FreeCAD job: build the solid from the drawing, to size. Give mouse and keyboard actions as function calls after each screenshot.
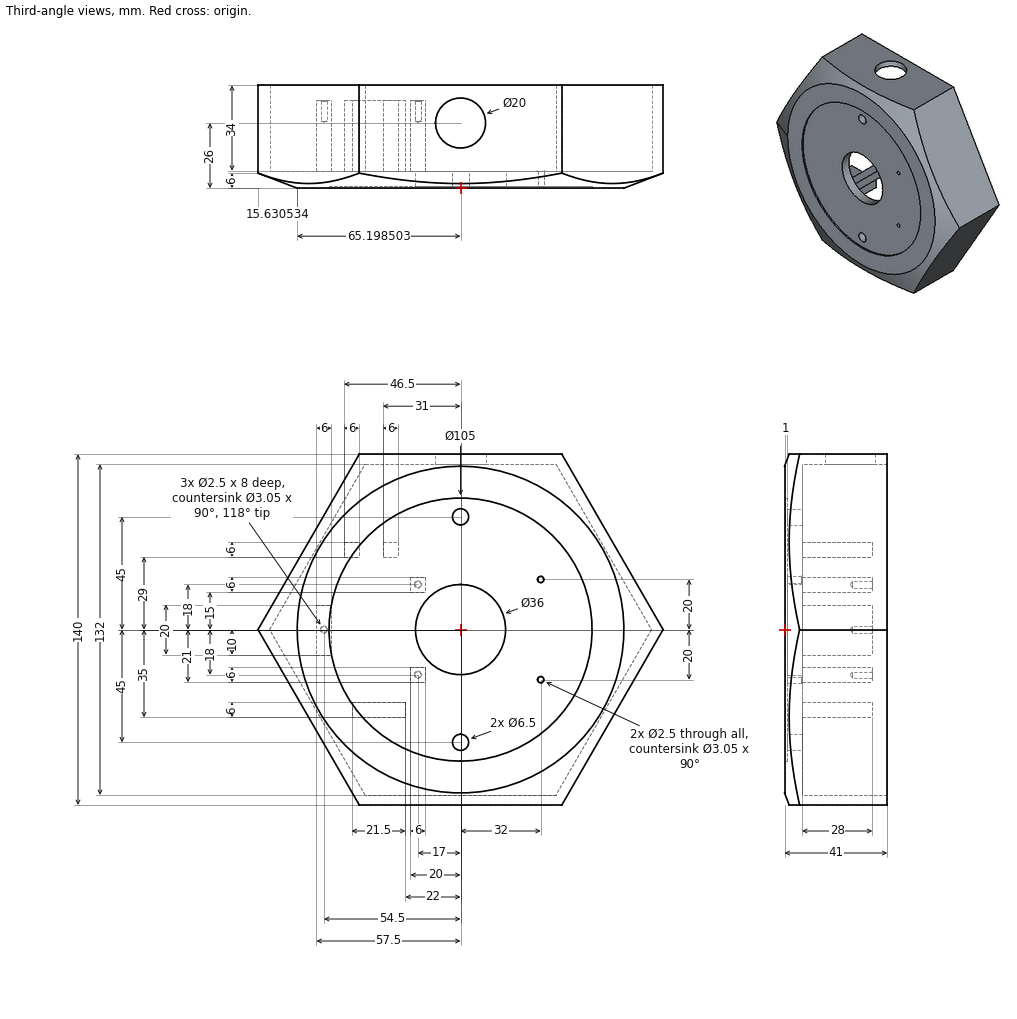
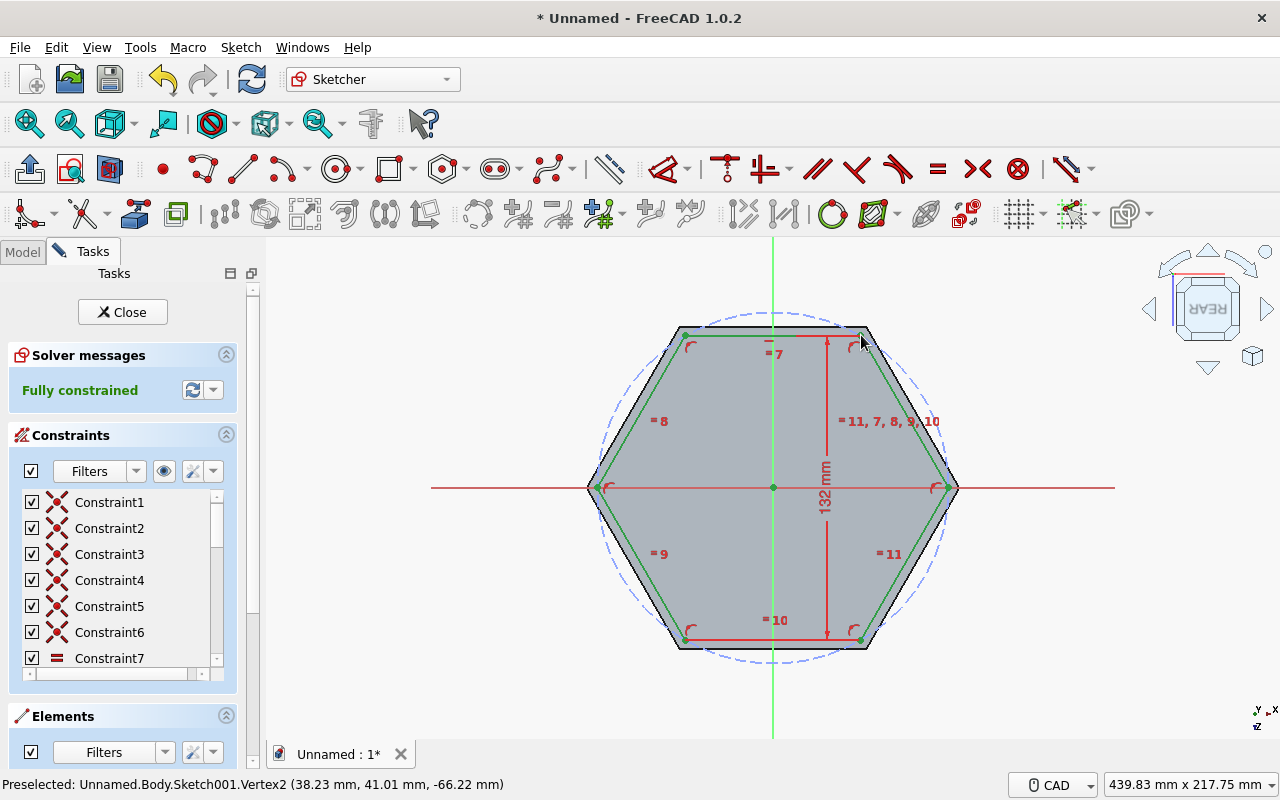
click(123, 312)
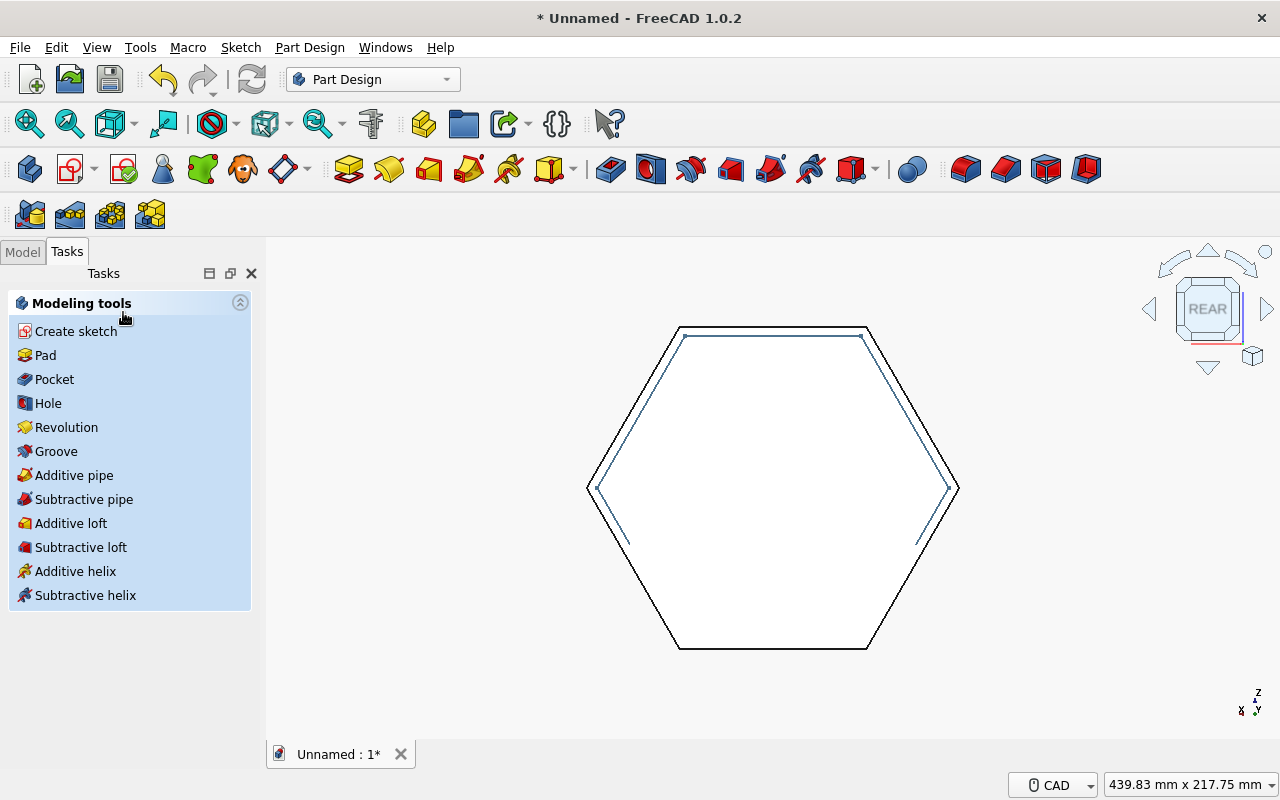
click(612, 170)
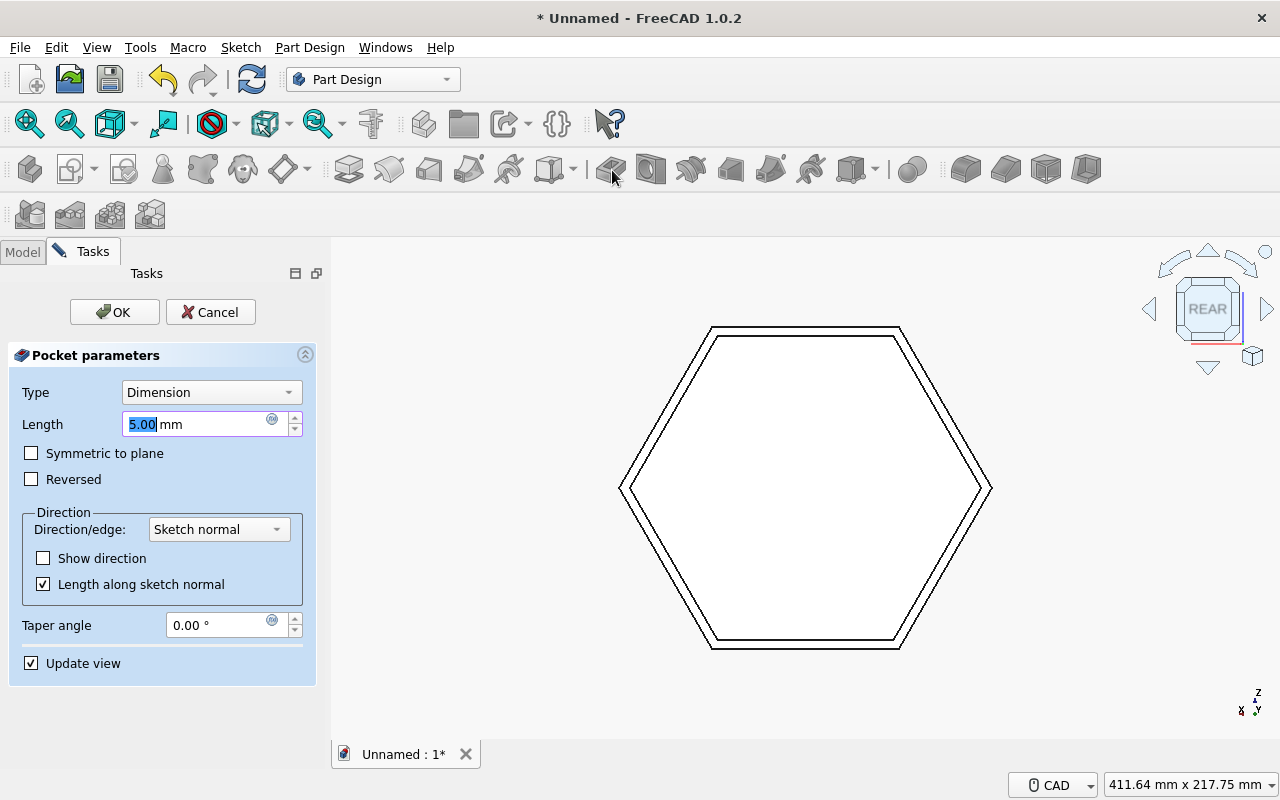
text(34)
key(Tab)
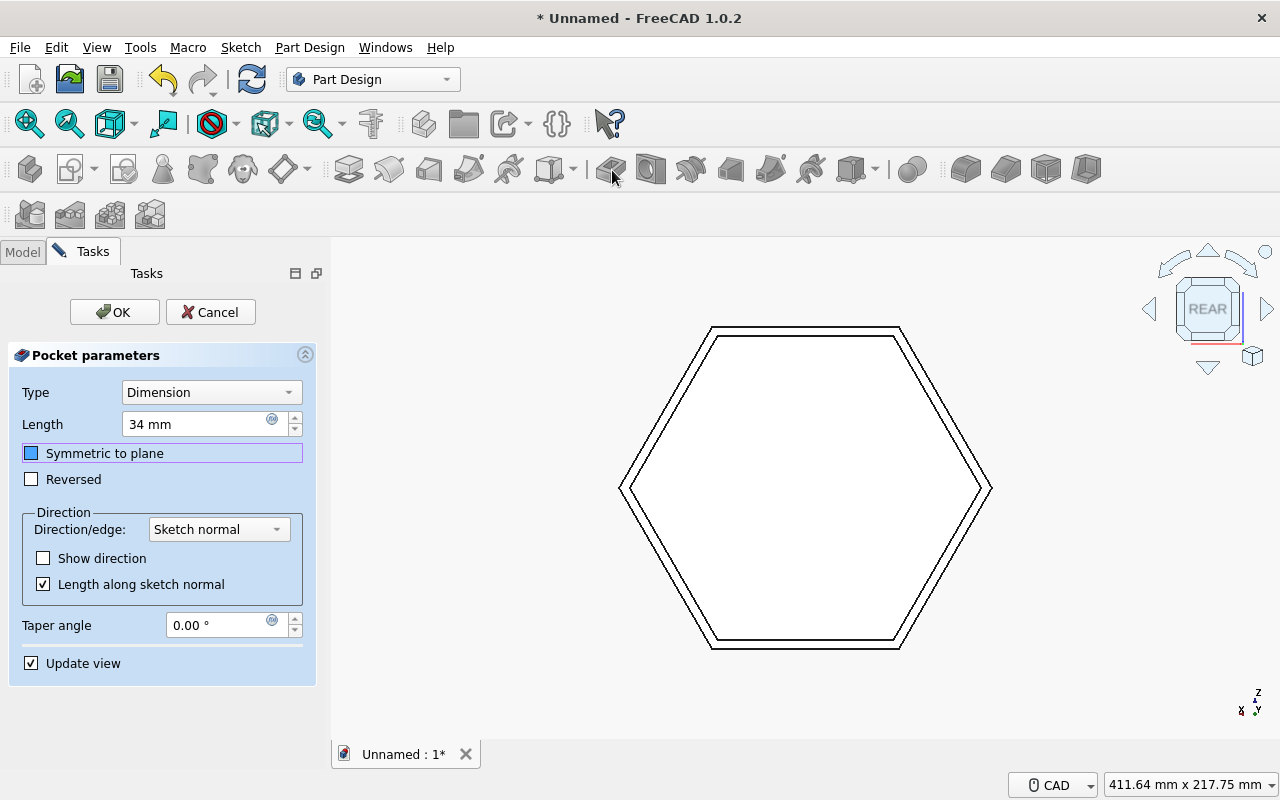
click(115, 312)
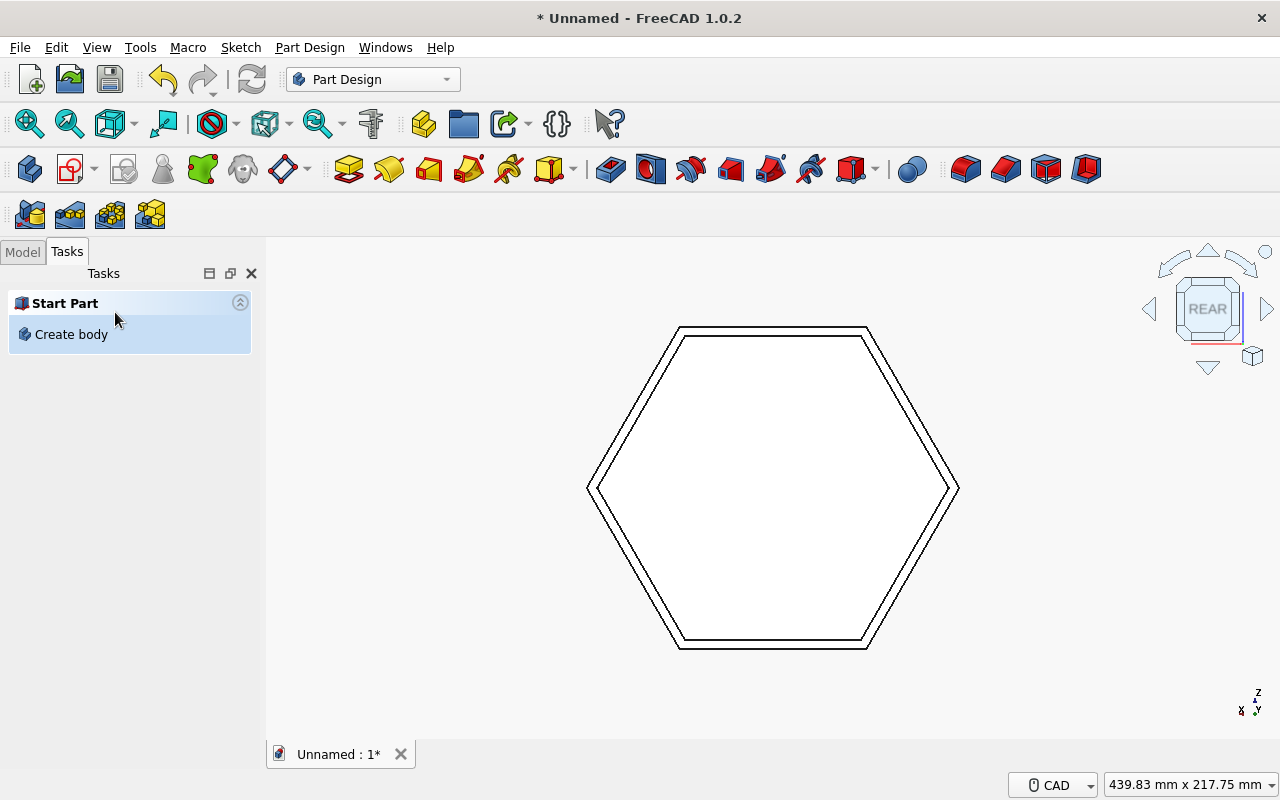
click(70, 170)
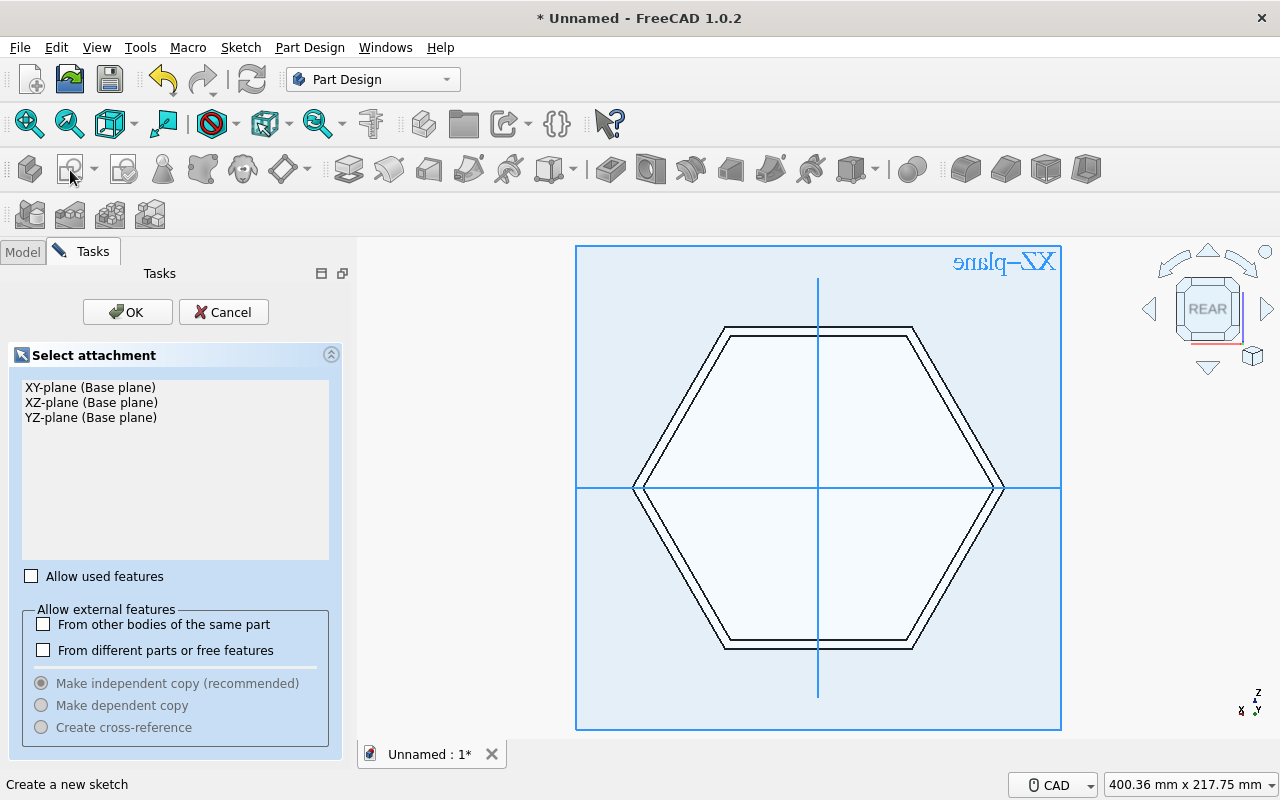
click(82, 388)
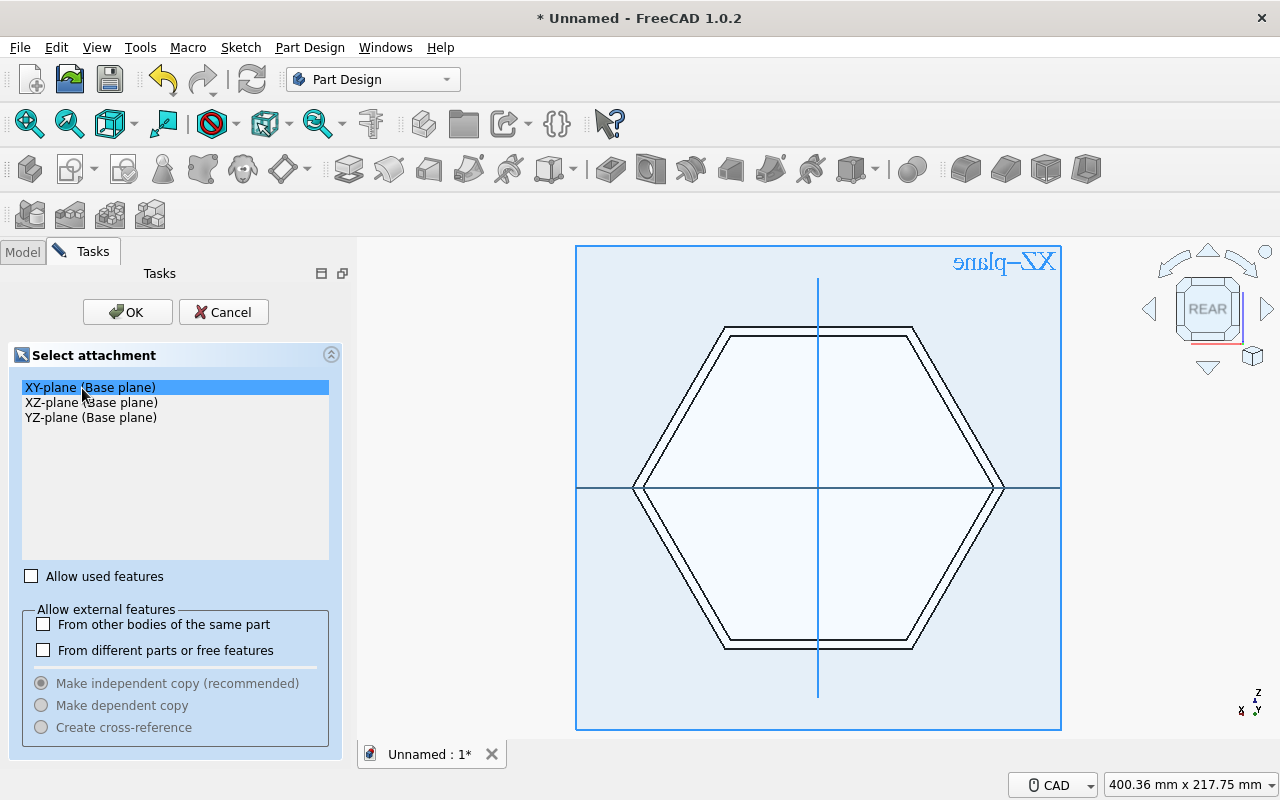
click(128, 312)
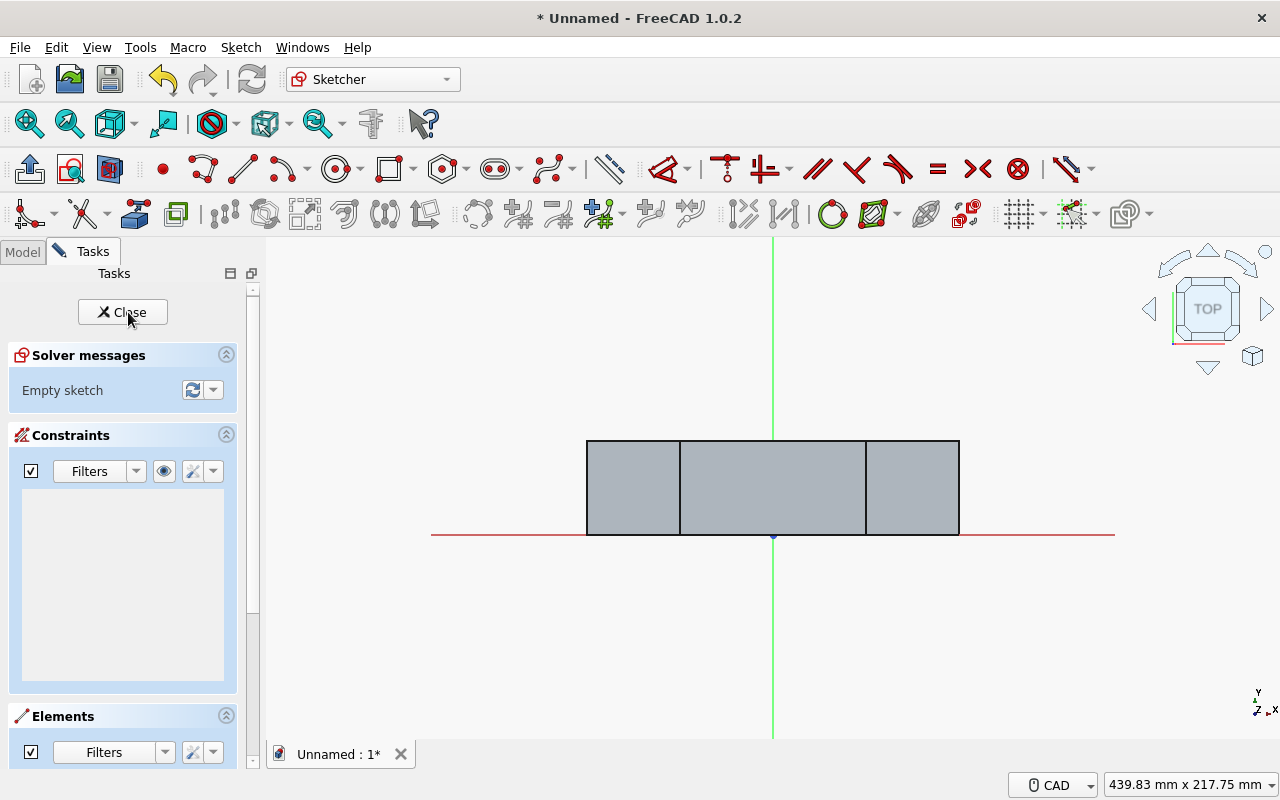
click(110, 170)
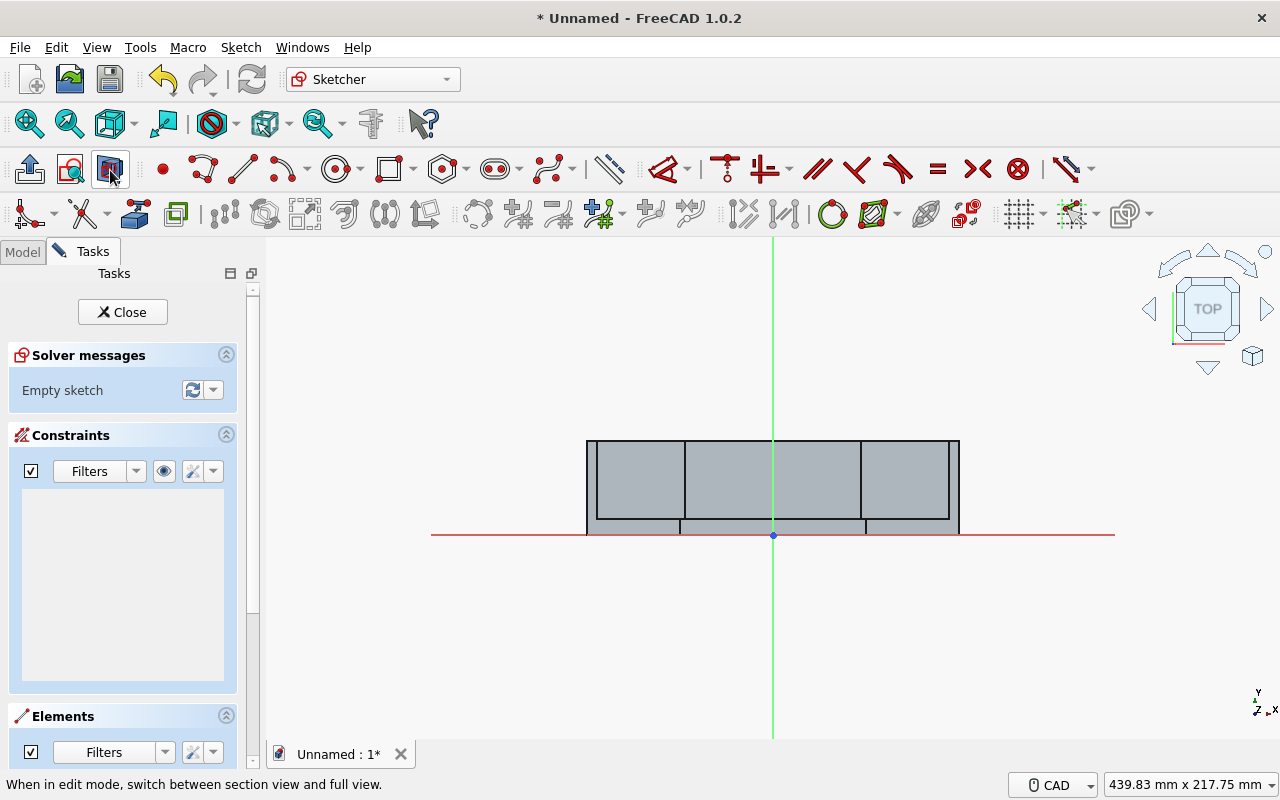
scroll(598, 531, up, 14)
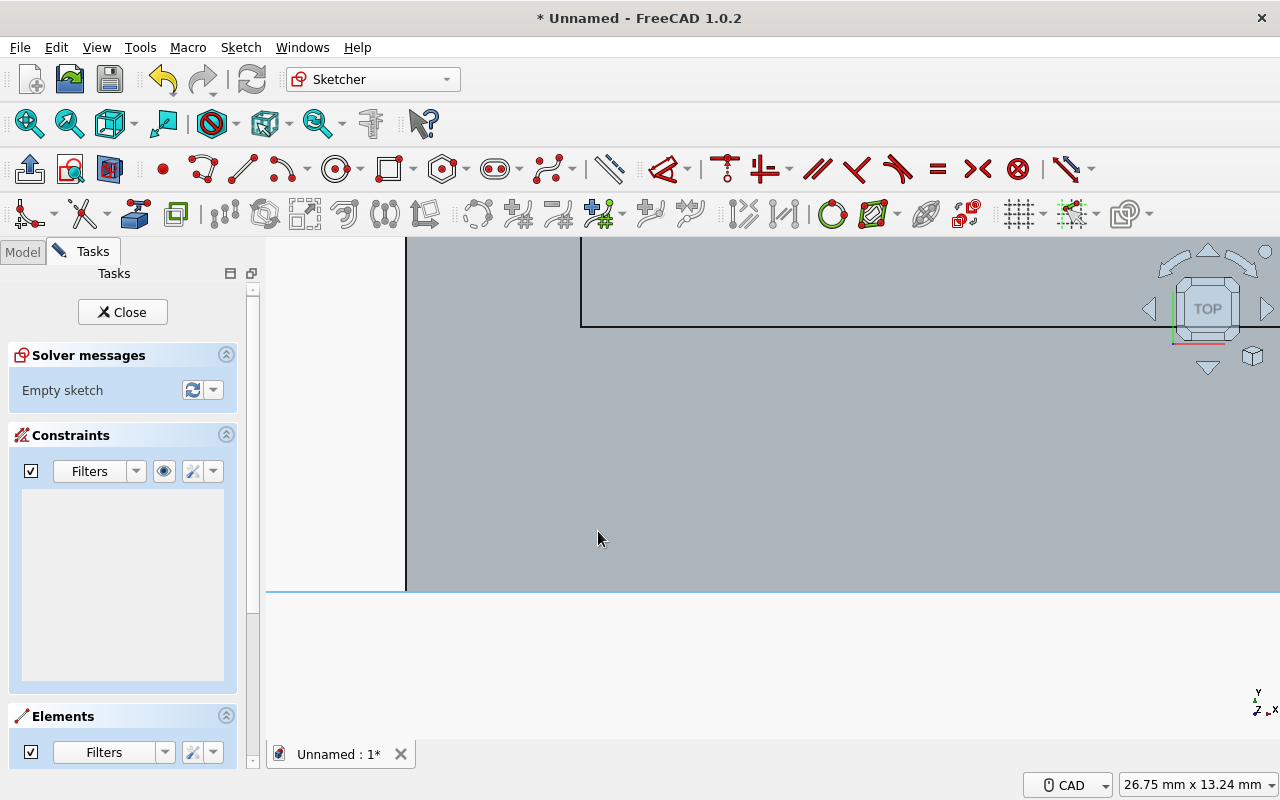
key(g)
key(m)